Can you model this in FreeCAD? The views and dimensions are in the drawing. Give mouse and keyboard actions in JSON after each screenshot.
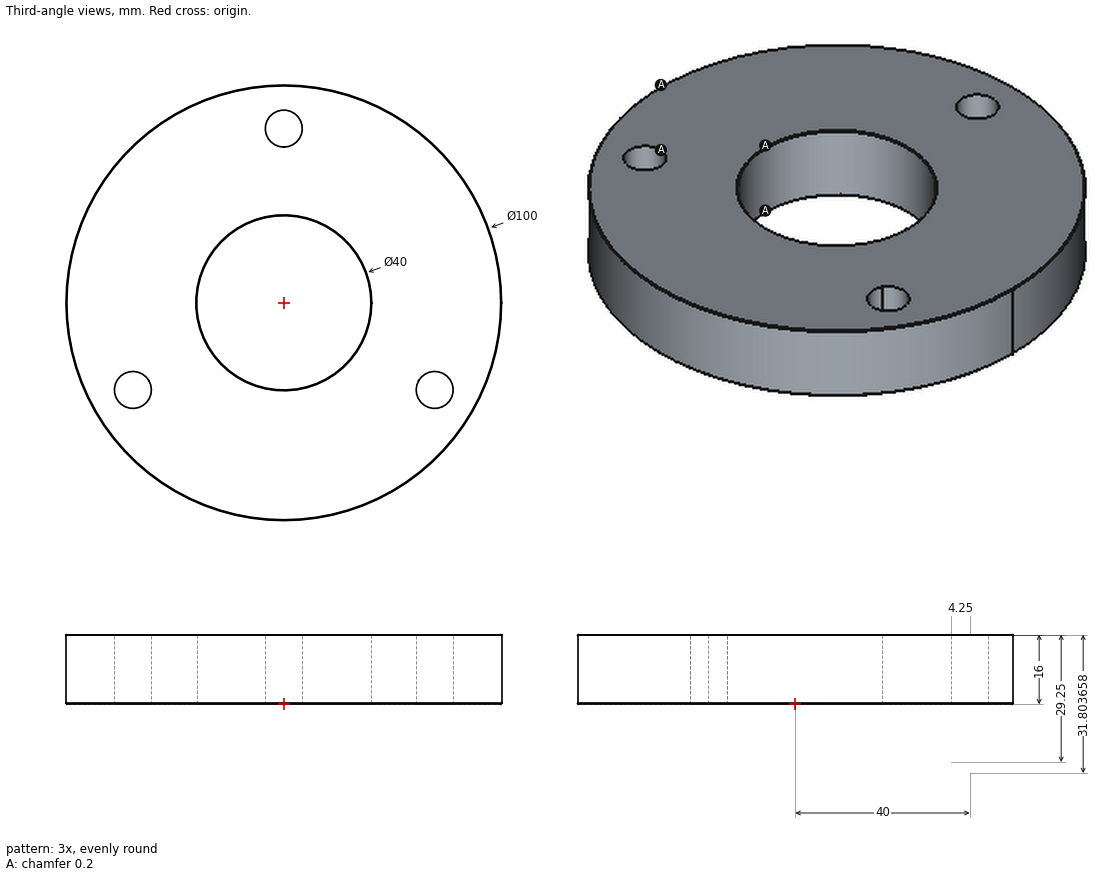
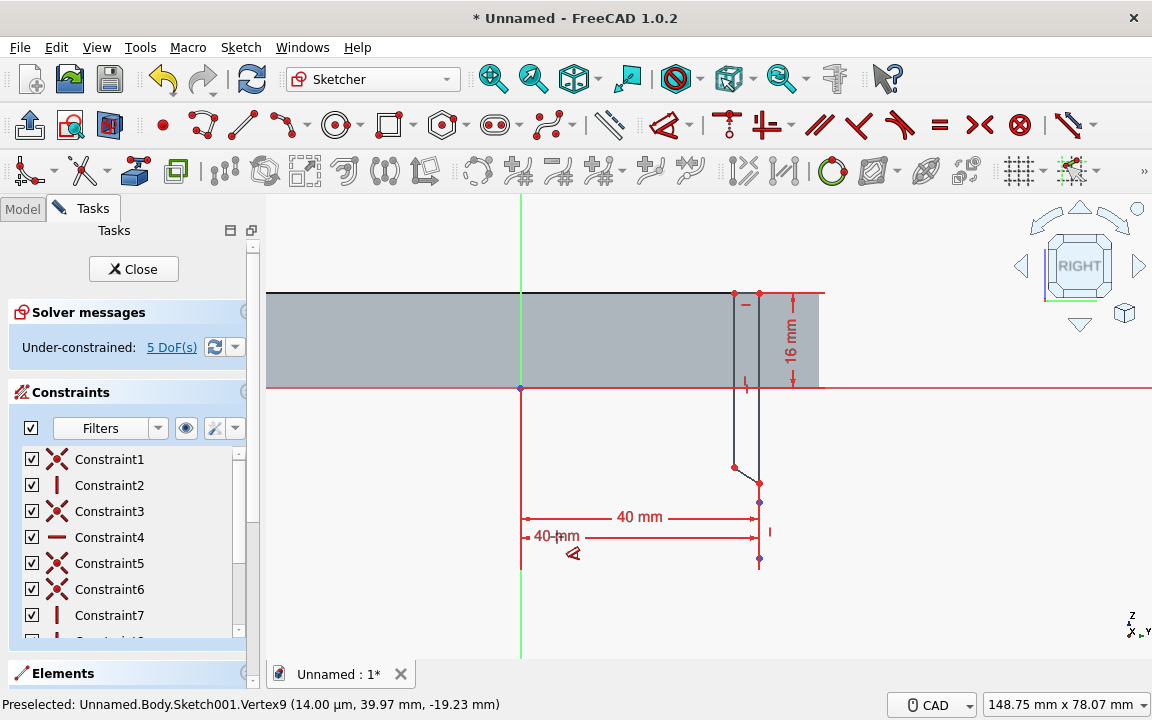
{"action": "scroll", "coordinate": [749, 293], "scroll_direction": "up", "scroll_amount": 3}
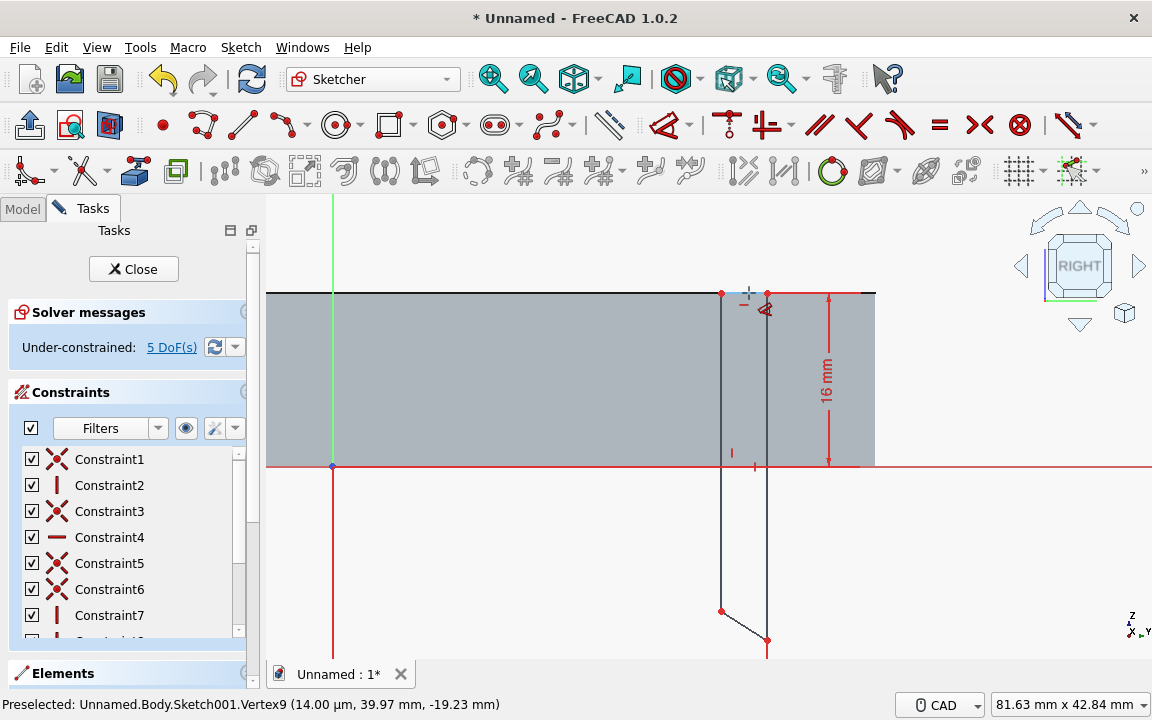
{"action": "left_click", "coordinate": [749, 293]}
{"action": "left_click", "coordinate": [744, 259]}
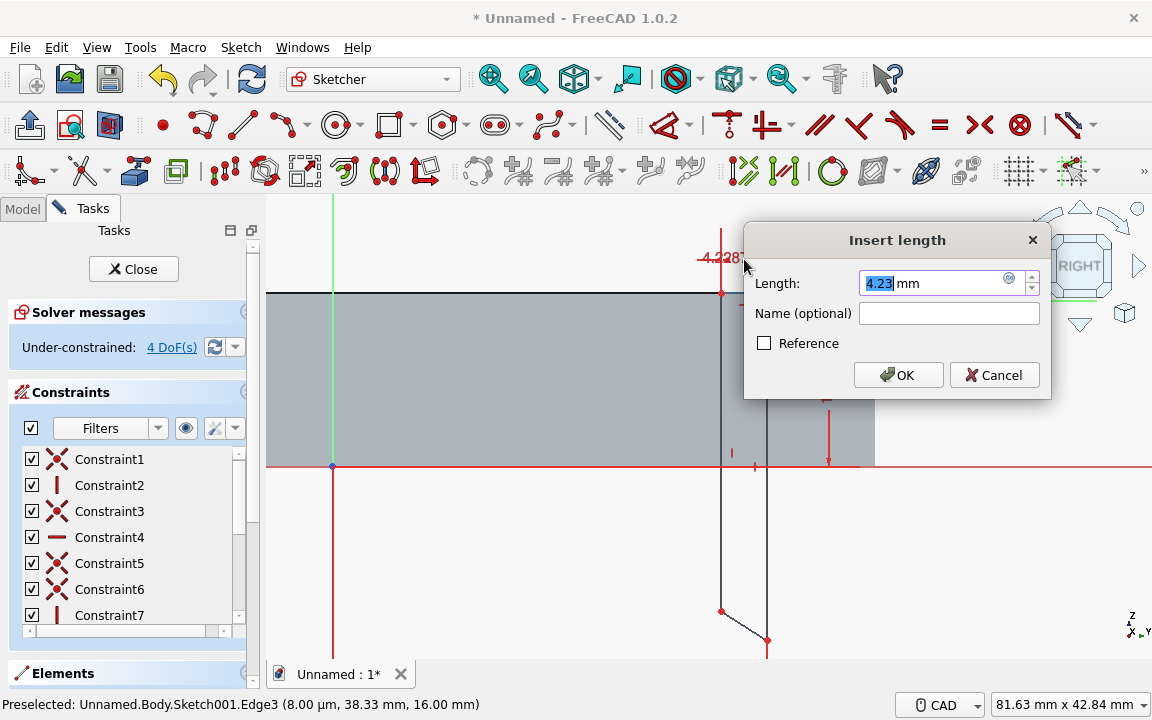
{"action": "type", "text": "4.25"}
{"action": "key", "text": "Return"}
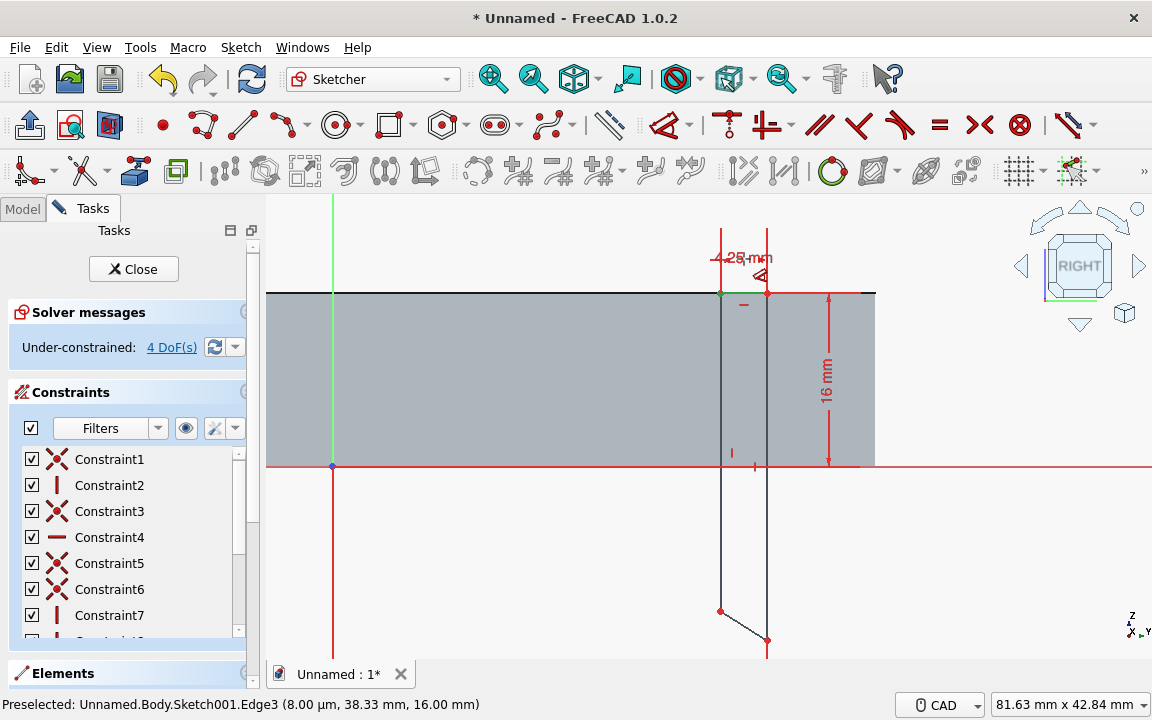
{"action": "left_click", "coordinate": [721, 389]}
{"action": "left_click", "coordinate": [687, 452]}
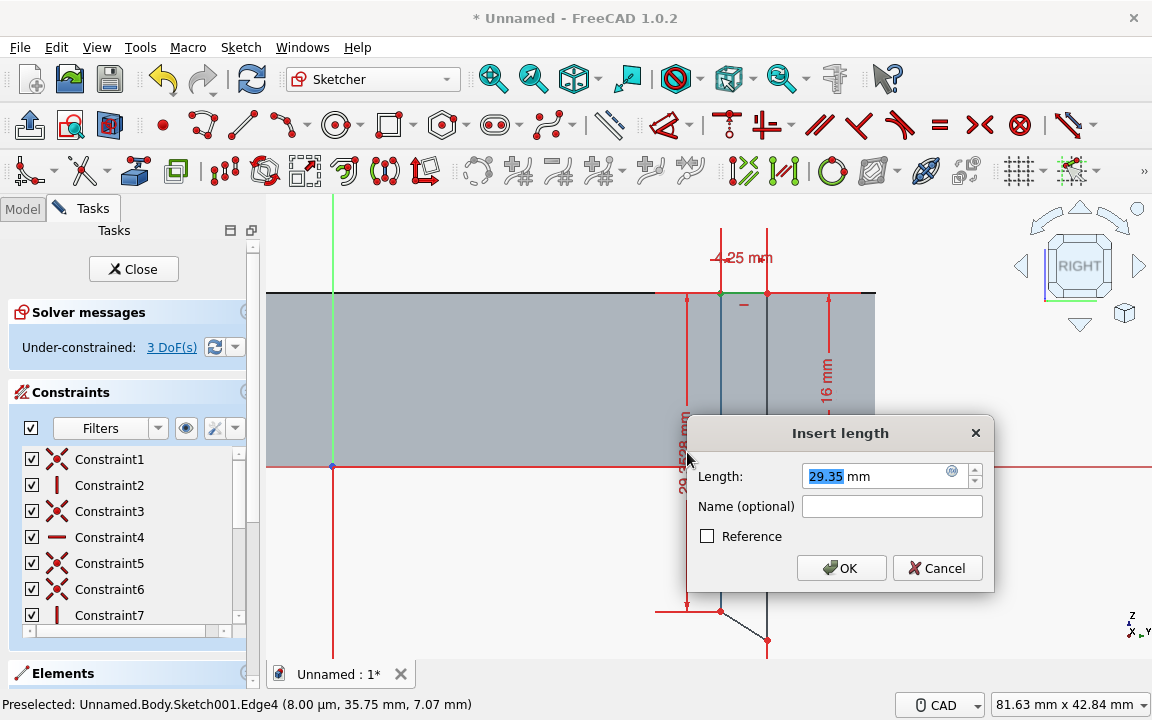
{"action": "type", "text": "29.25"}
{"action": "key", "text": "Return"}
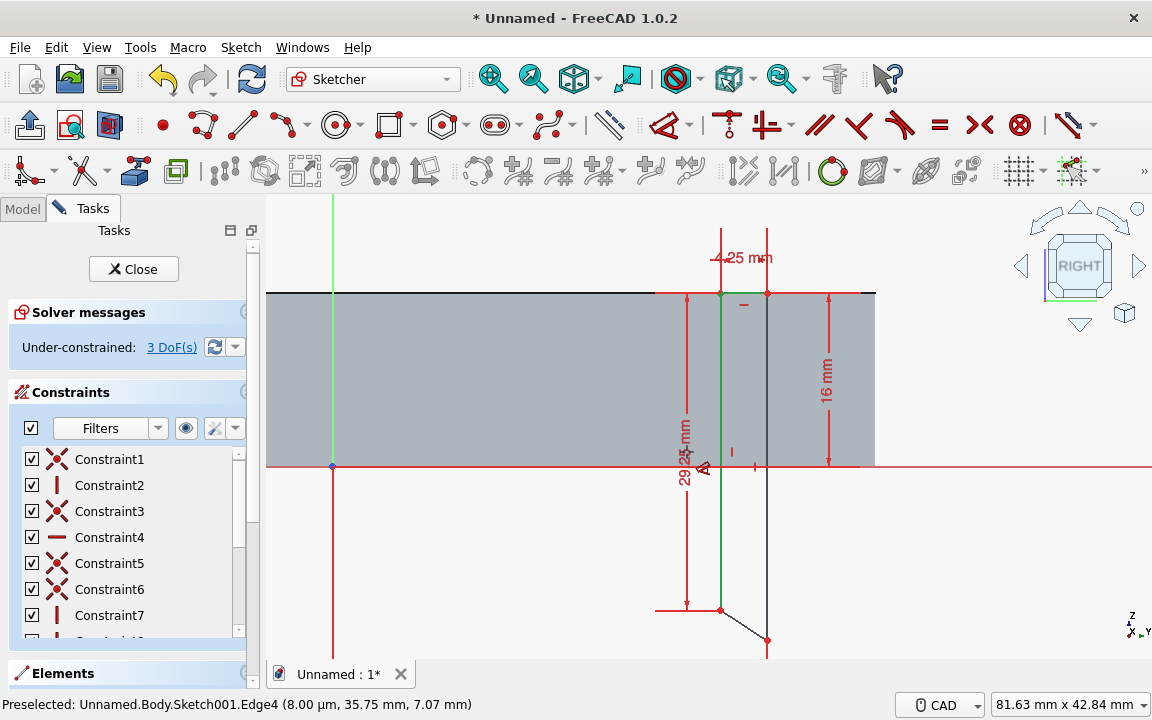
{"action": "left_click", "coordinate": [767, 537]}
{"action": "left_click", "coordinate": [801, 540]}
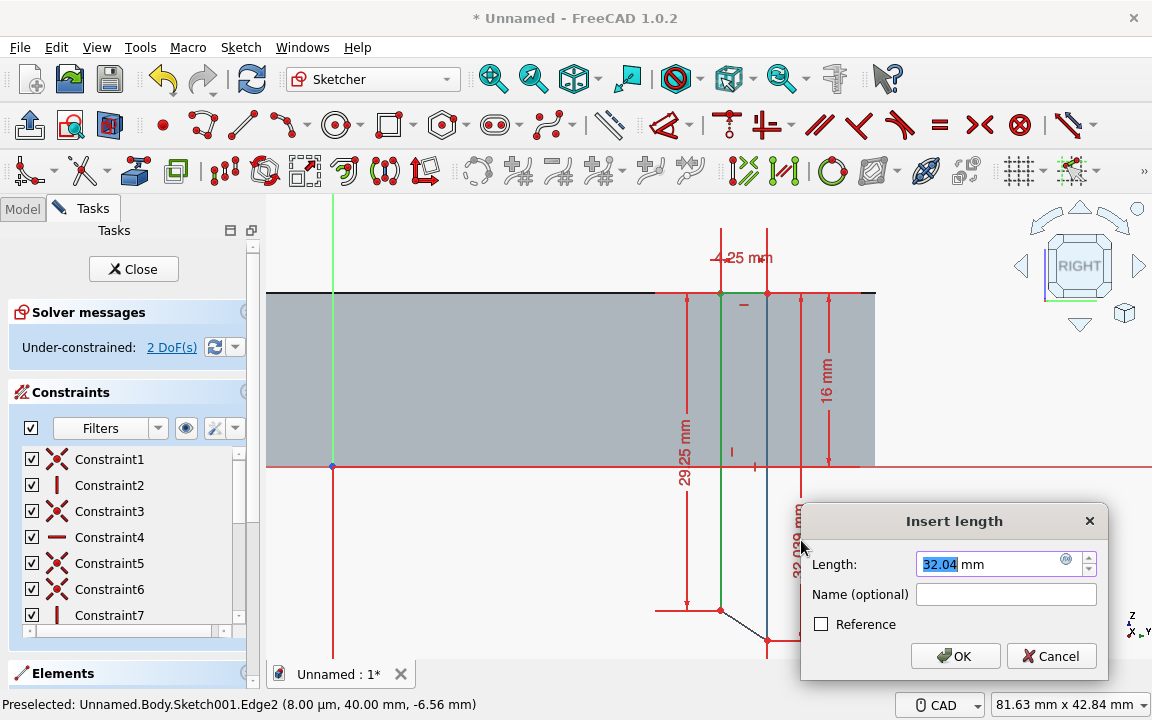
{"action": "type", "text": "31.803658"}
{"action": "key", "text": "Return"}
{"action": "key", "text": "Escape"}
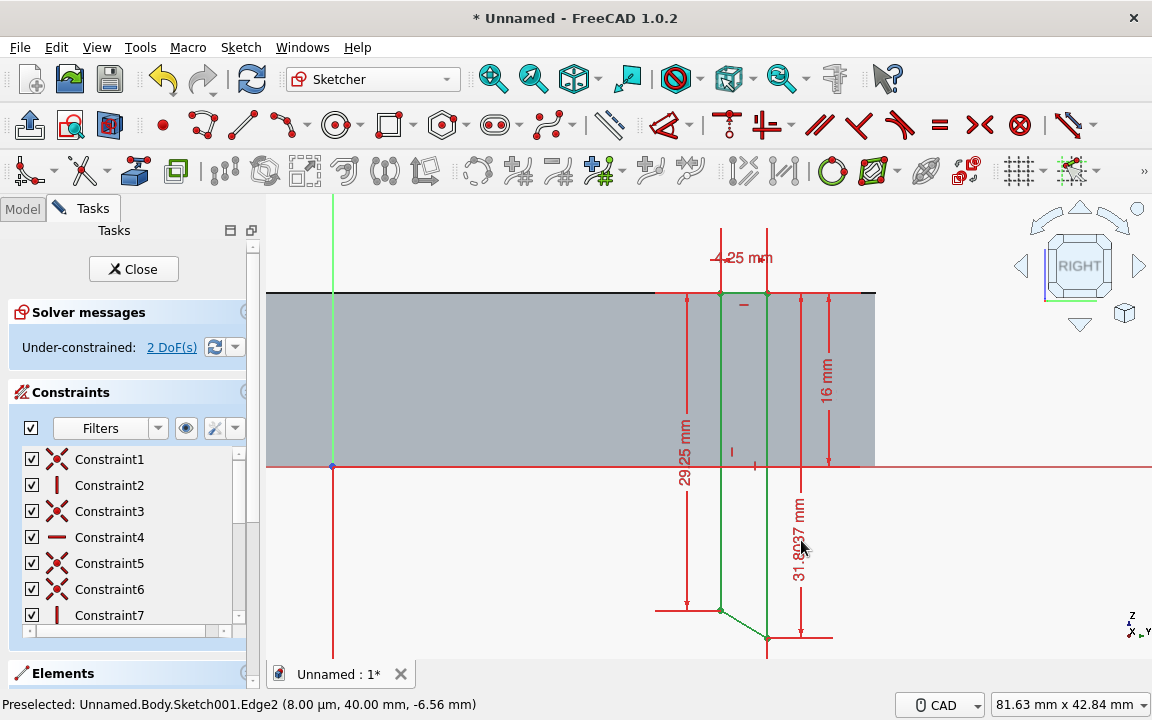
{"action": "left_click", "coordinate": [134, 269]}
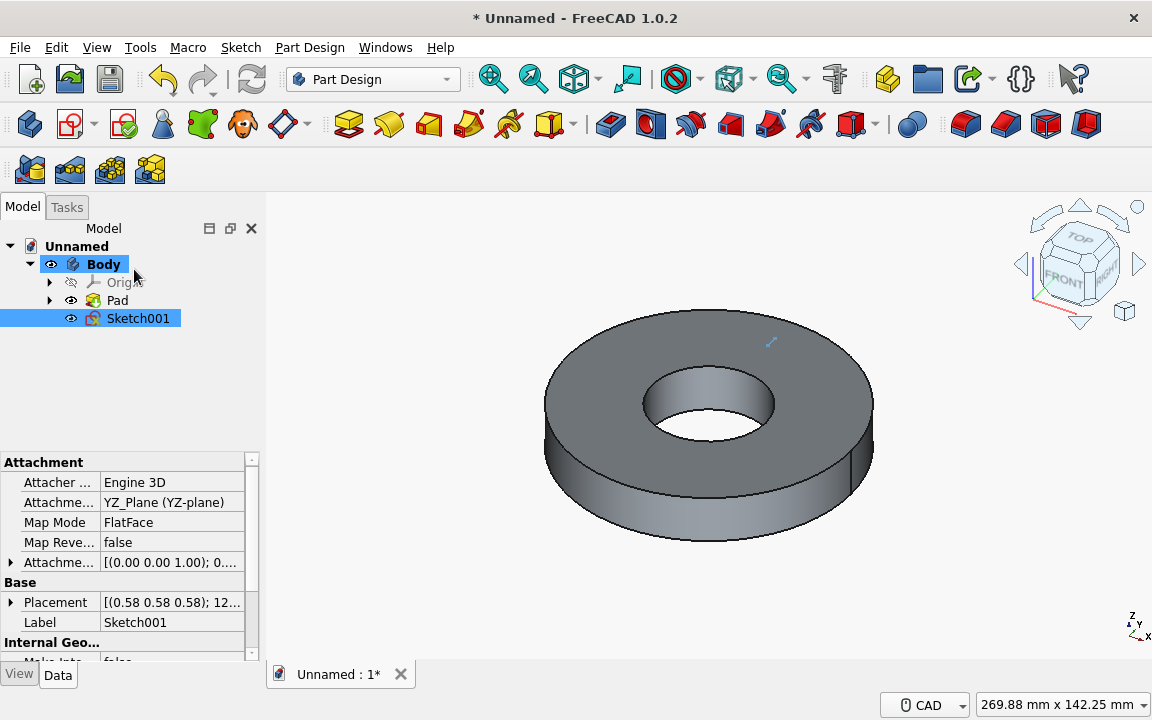
{"action": "left_click", "coordinate": [692, 124]}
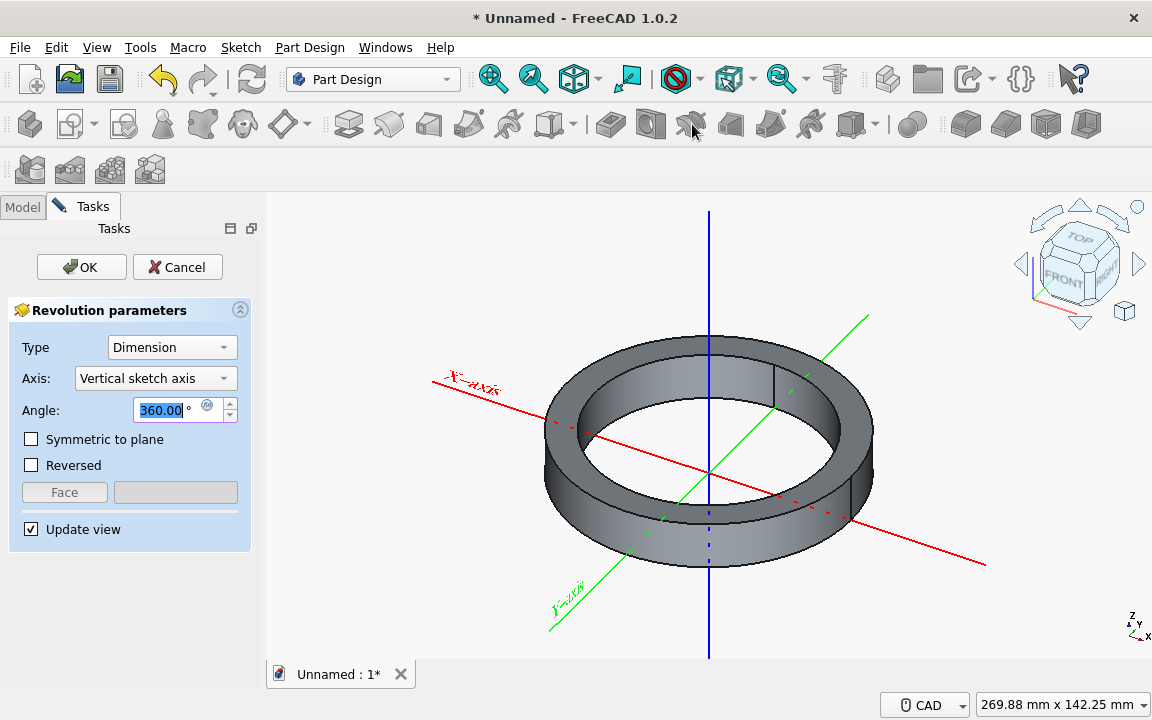
{"action": "left_click", "coordinate": [156, 378]}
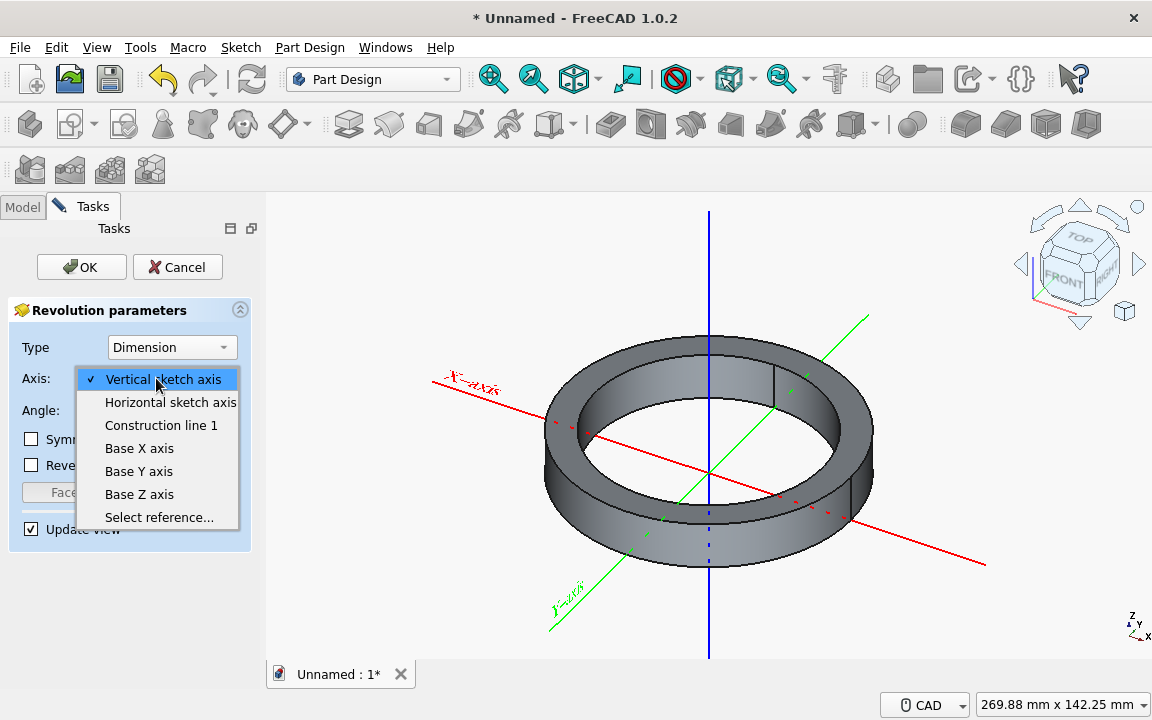
{"action": "left_click", "coordinate": [156, 426]}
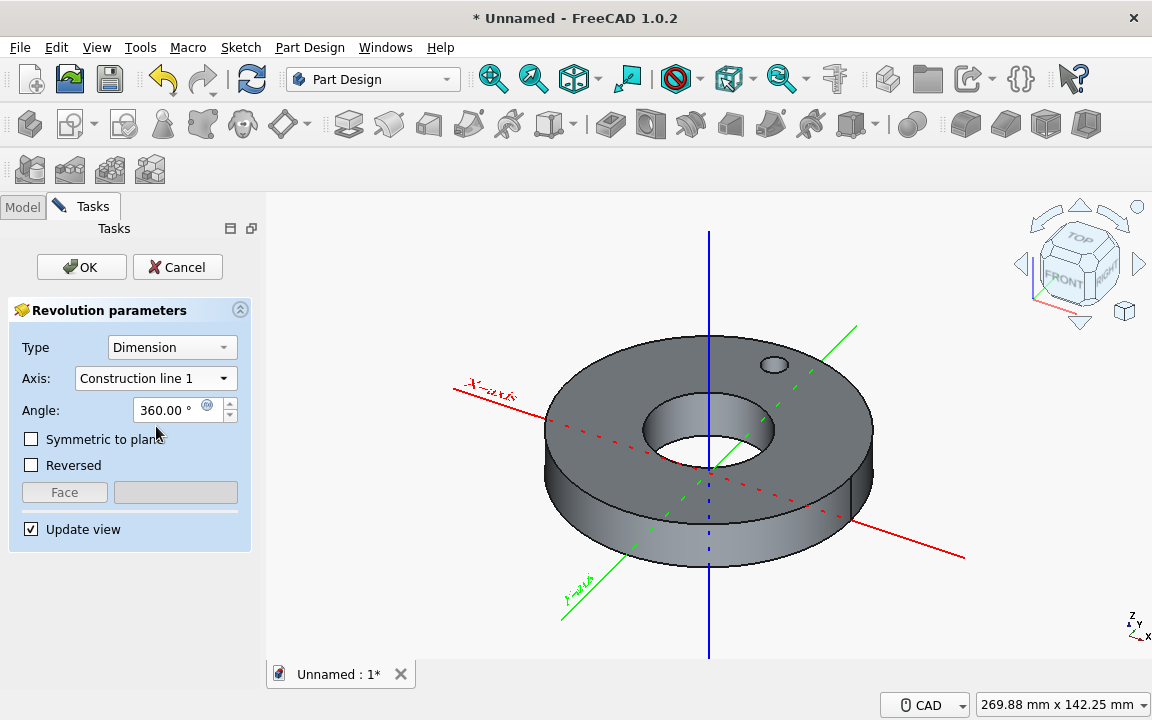
{"action": "left_click", "coordinate": [82, 267]}